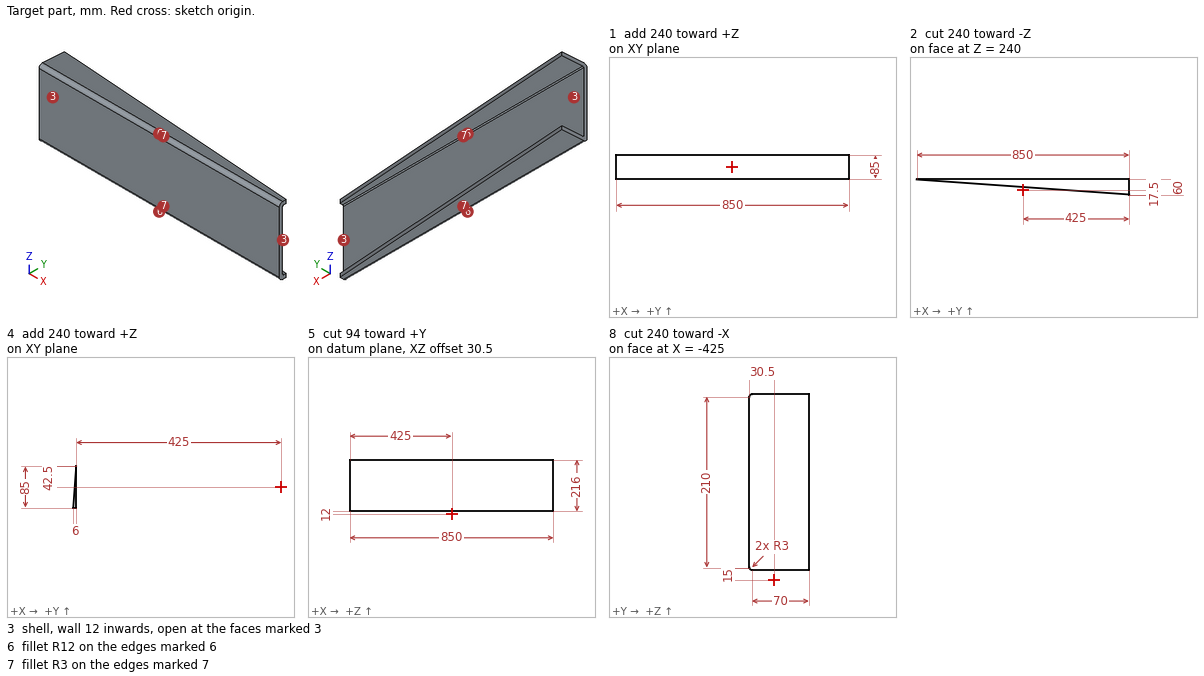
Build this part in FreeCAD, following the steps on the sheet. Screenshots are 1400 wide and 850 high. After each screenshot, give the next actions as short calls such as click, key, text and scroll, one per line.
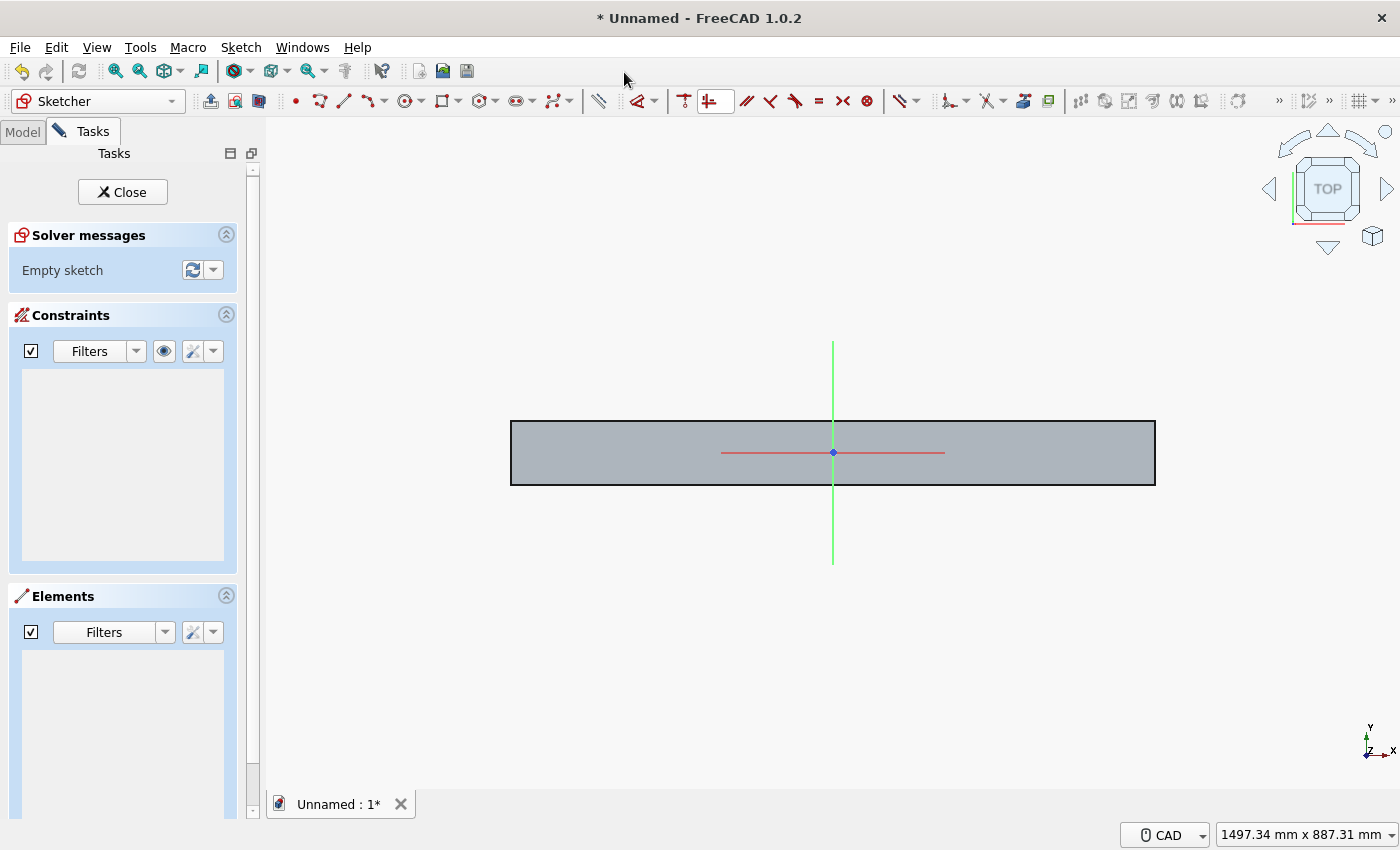
click(1155, 466)
click(1155, 421)
click(511, 421)
click(1155, 467)
key(Escape)
key(Escape)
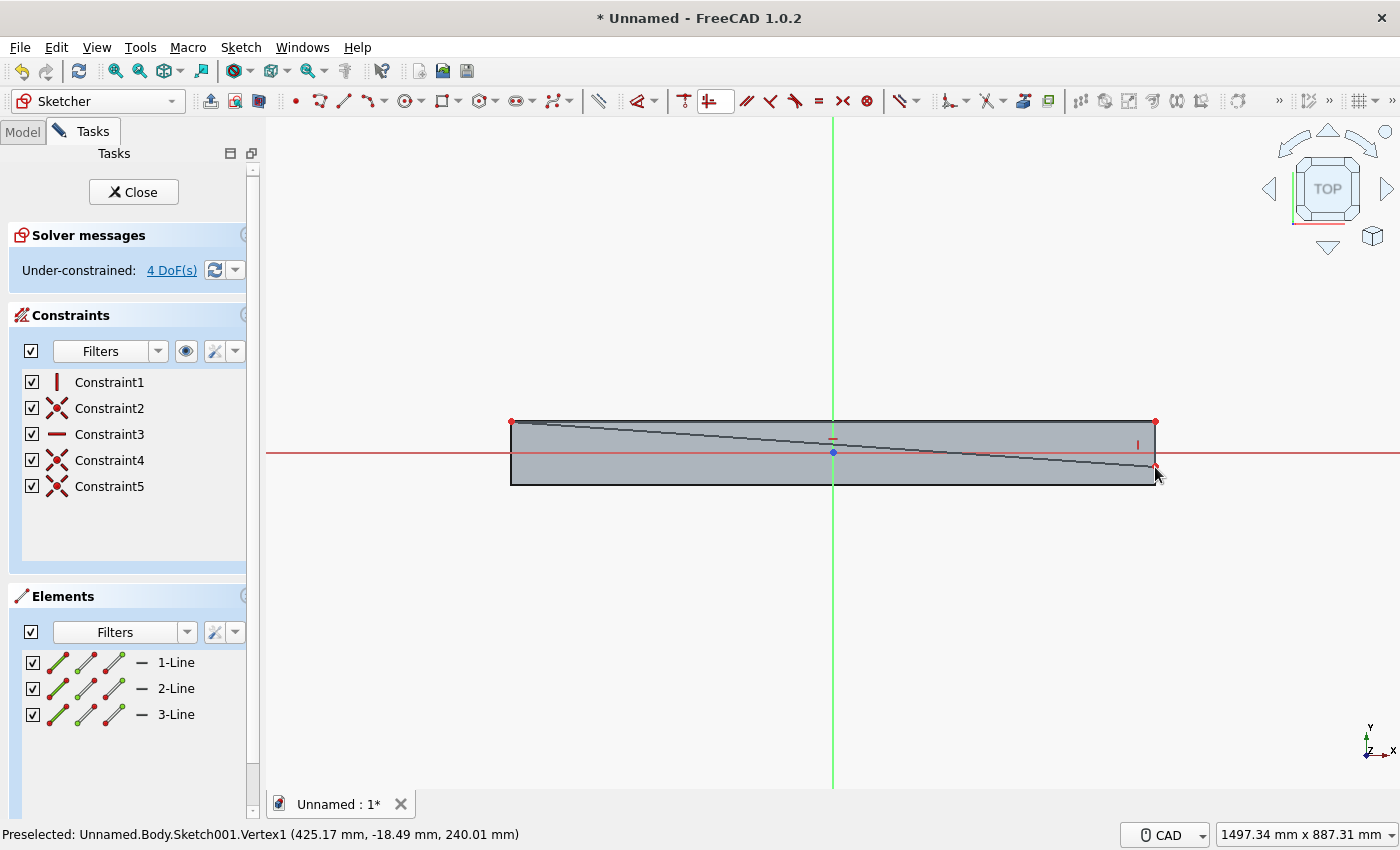
key(d)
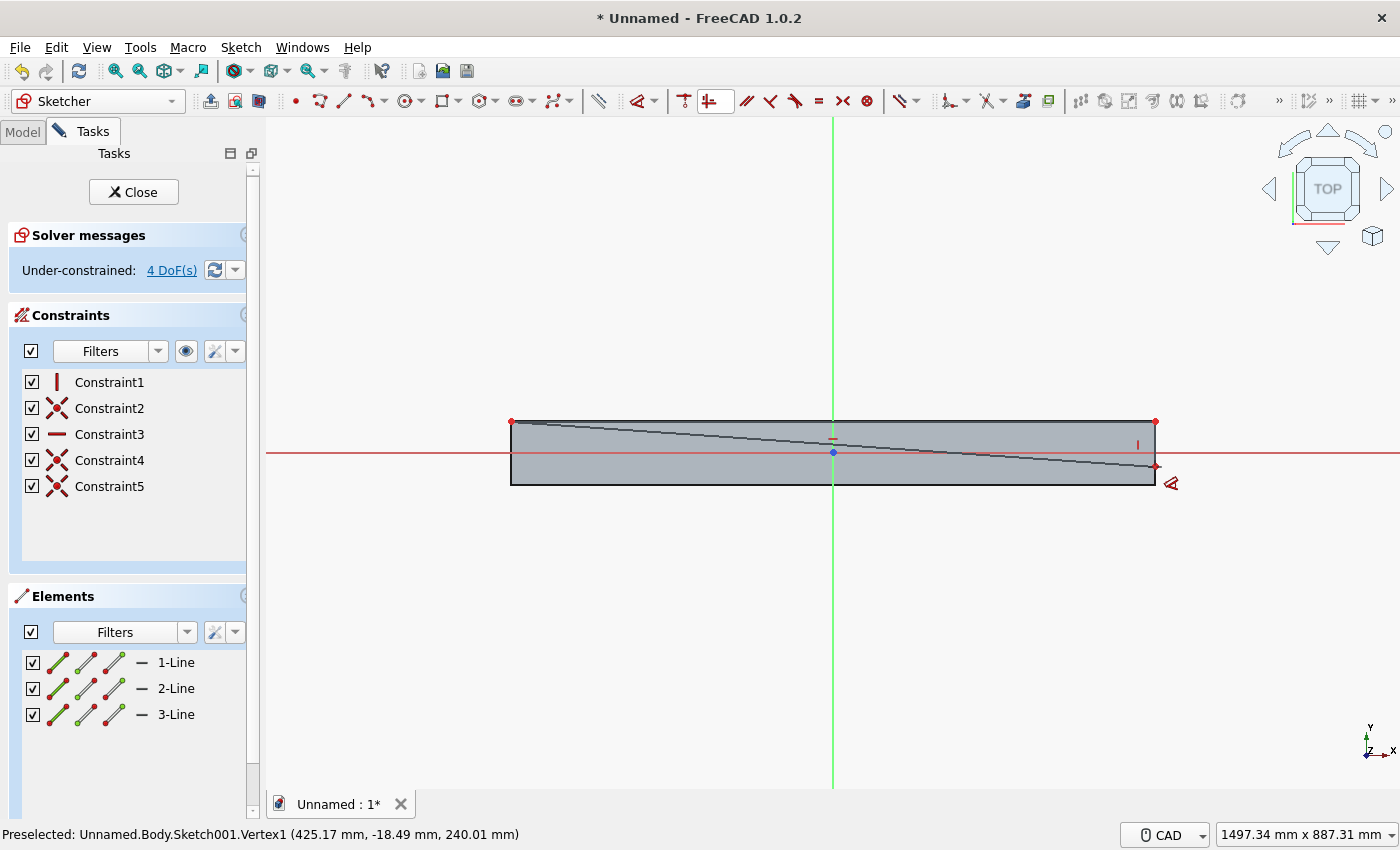
click(1155, 454)
click(1189, 434)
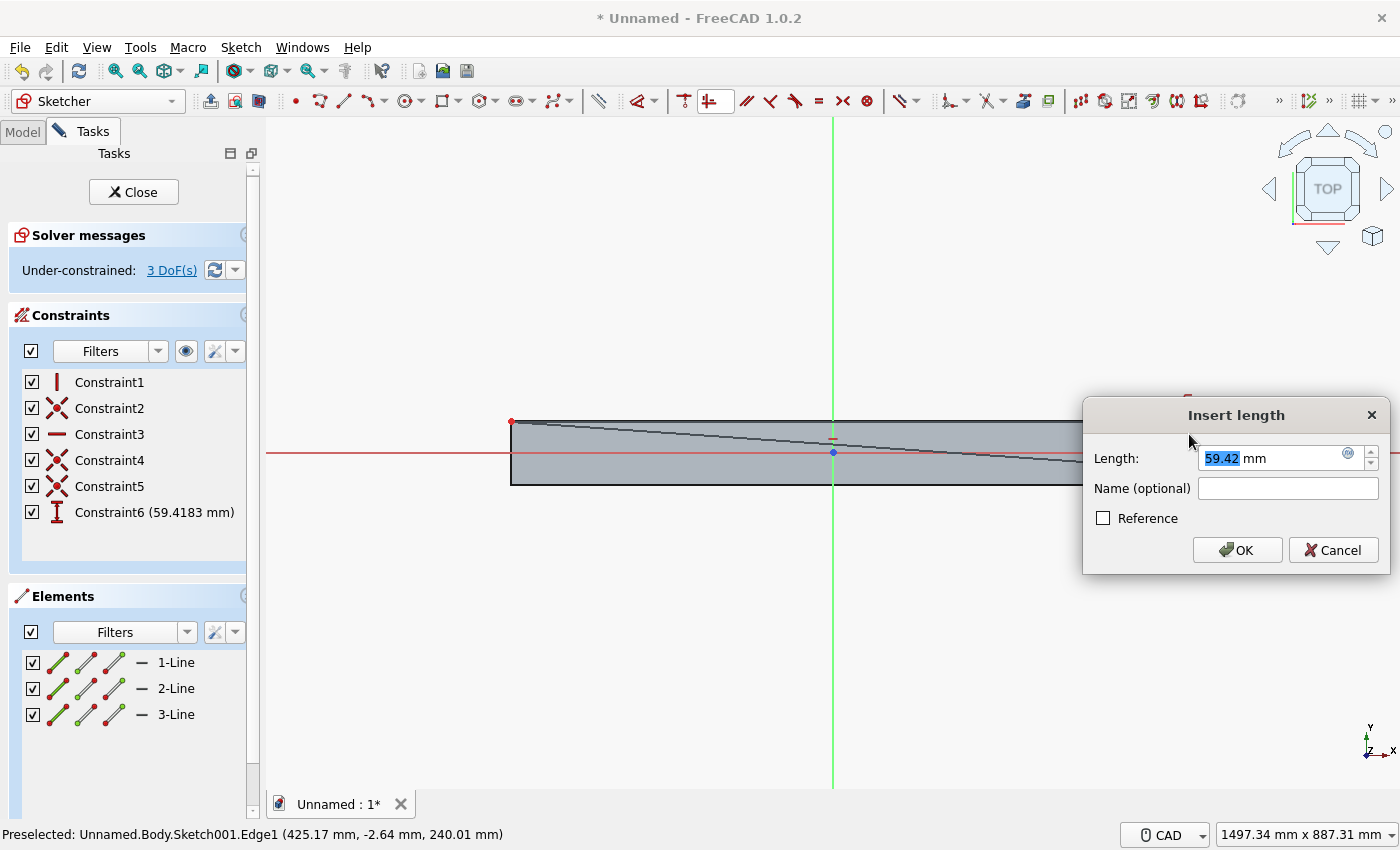
text(60)
key(Return)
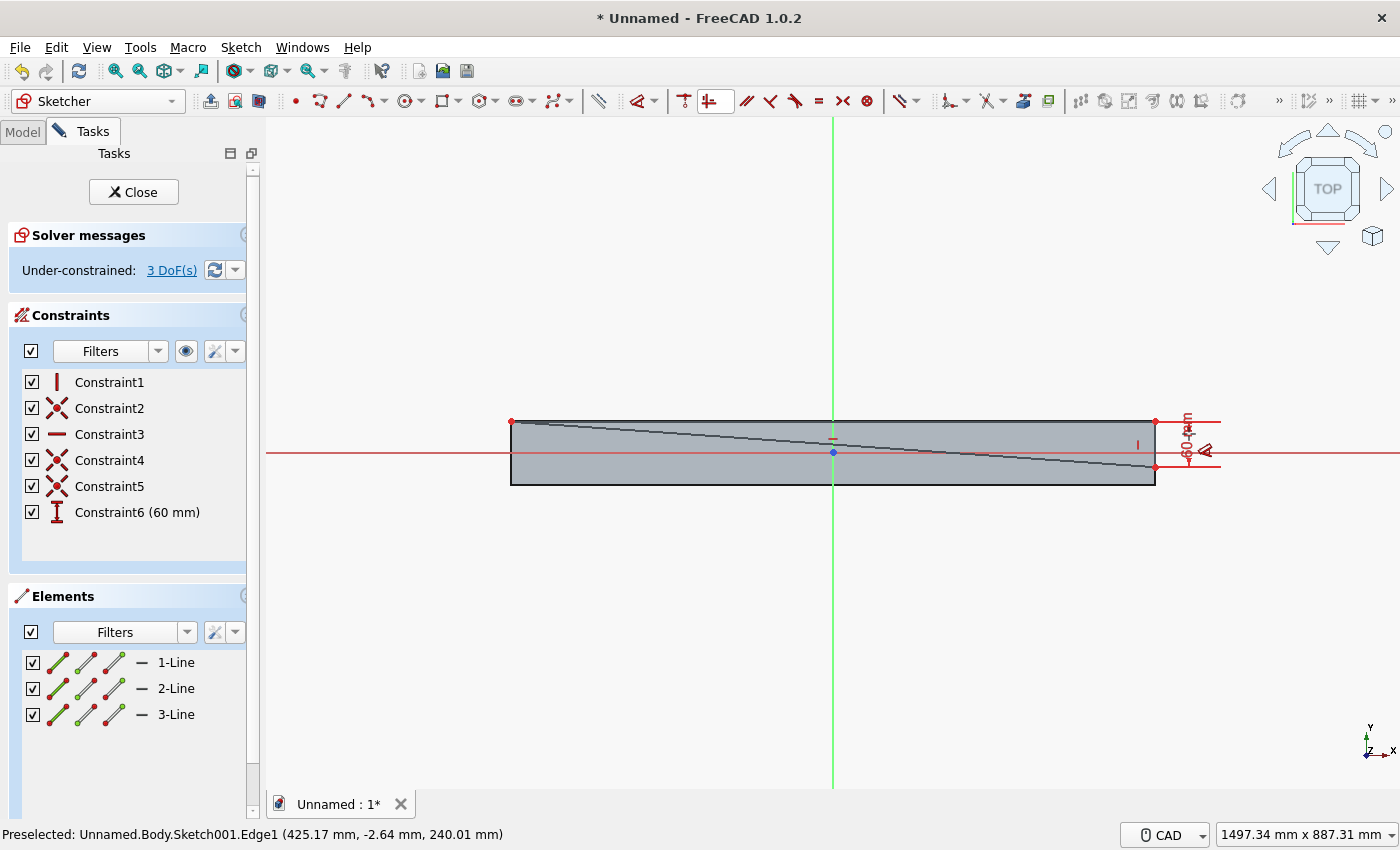
click(962, 422)
click(685, 388)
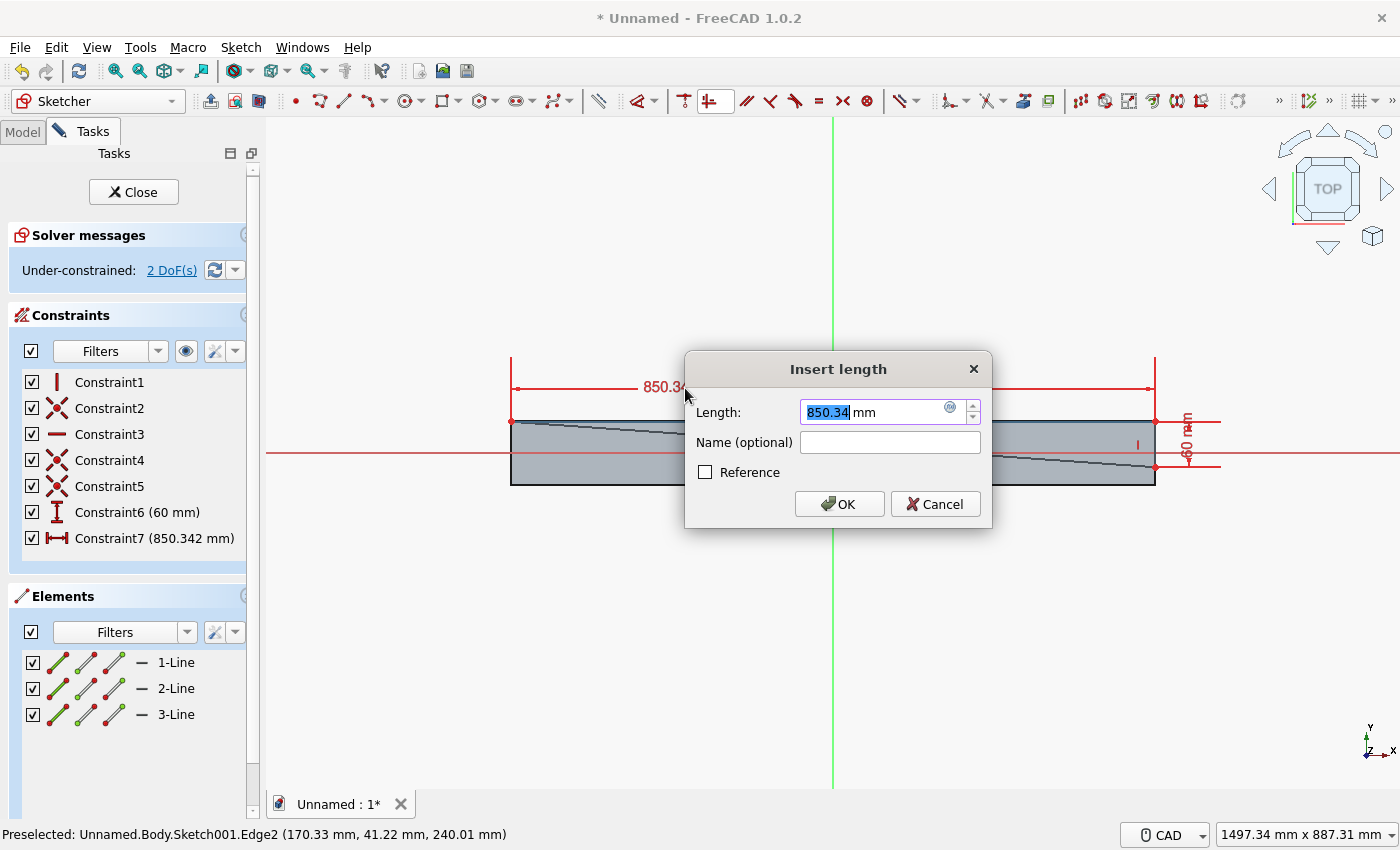
text(850)
key(Return)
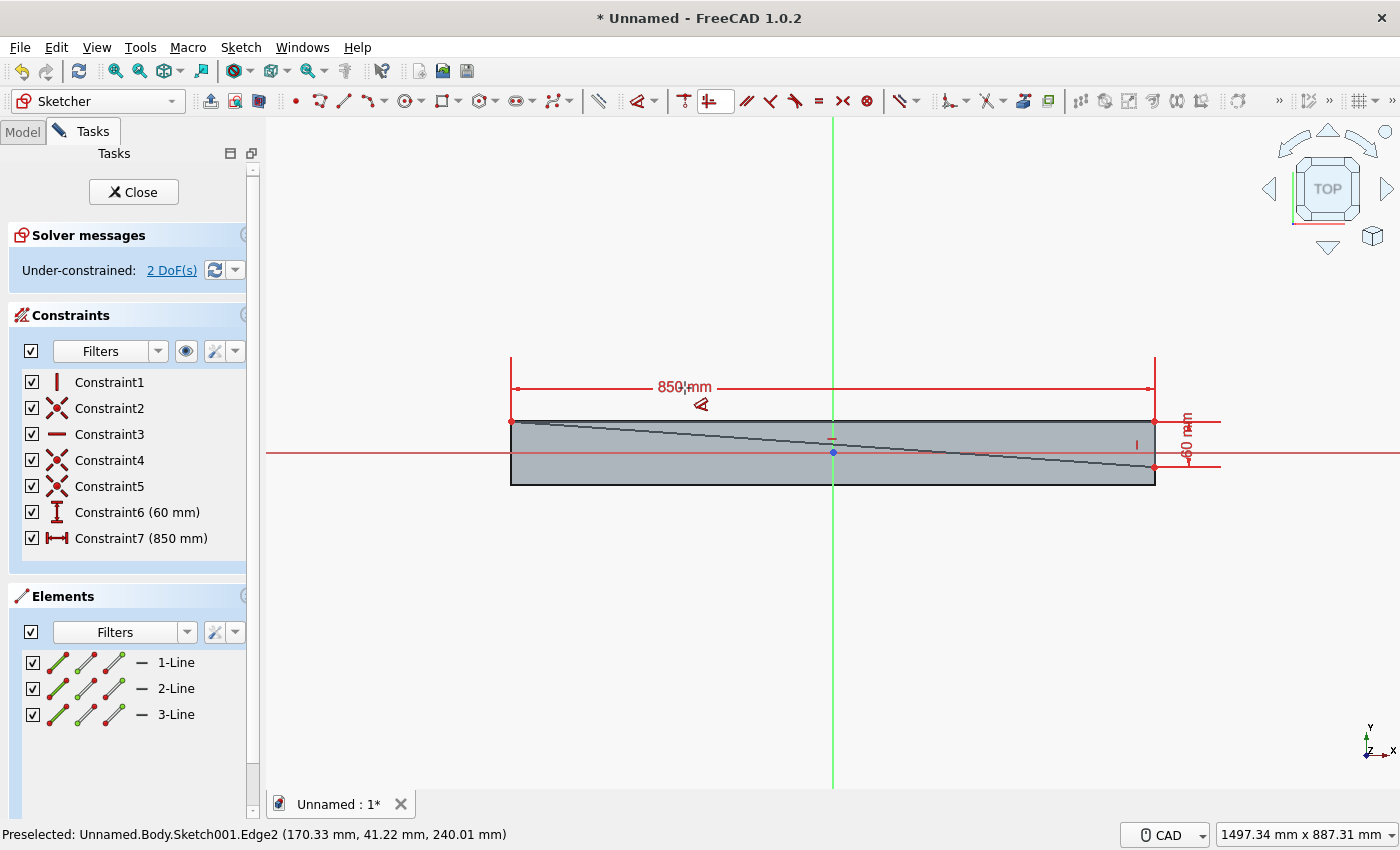
click(1155, 467)
click(994, 501)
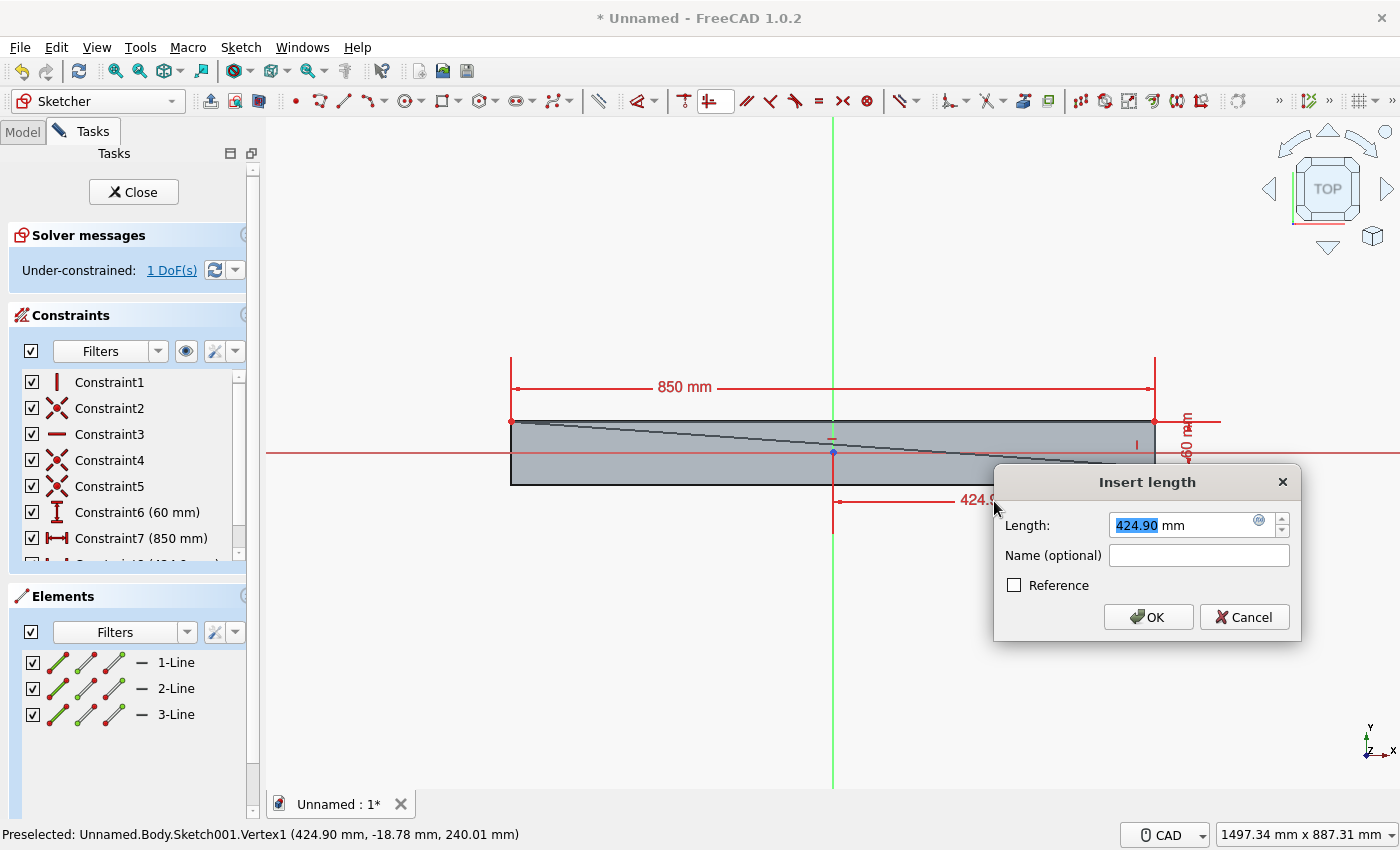
text(425)
key(Return)